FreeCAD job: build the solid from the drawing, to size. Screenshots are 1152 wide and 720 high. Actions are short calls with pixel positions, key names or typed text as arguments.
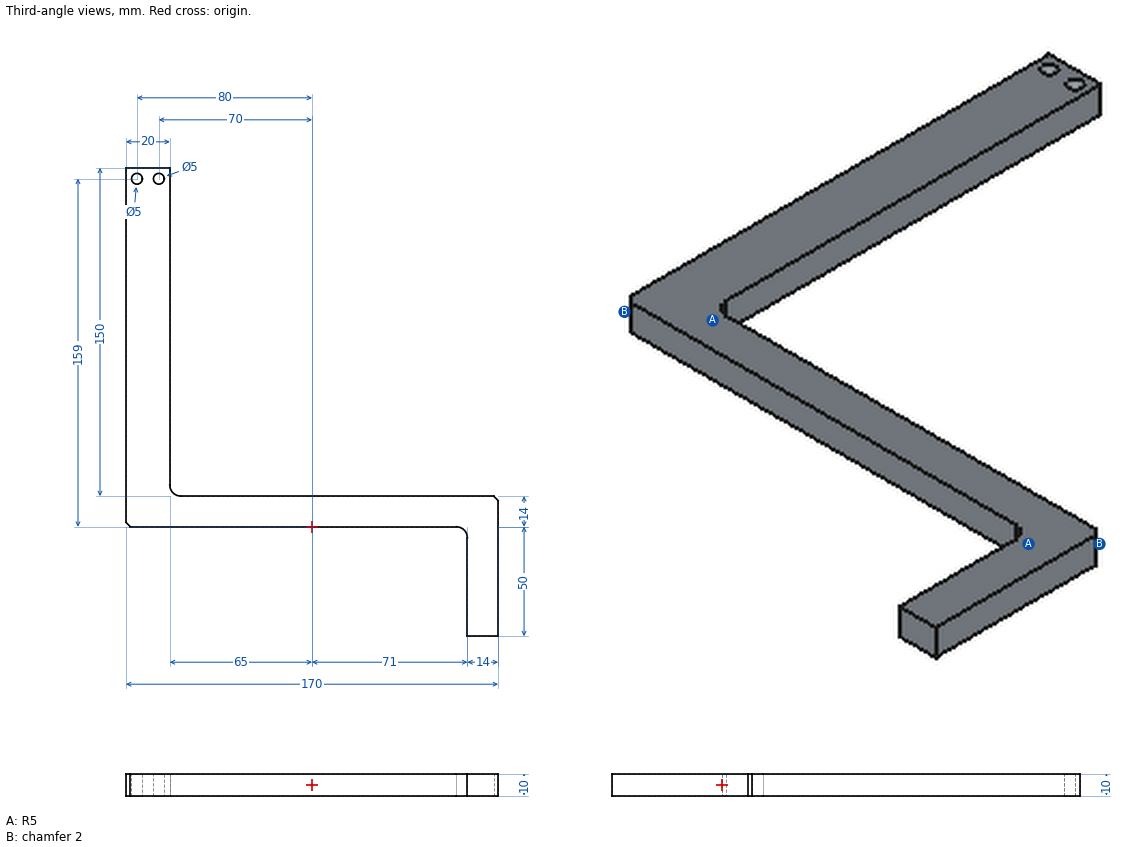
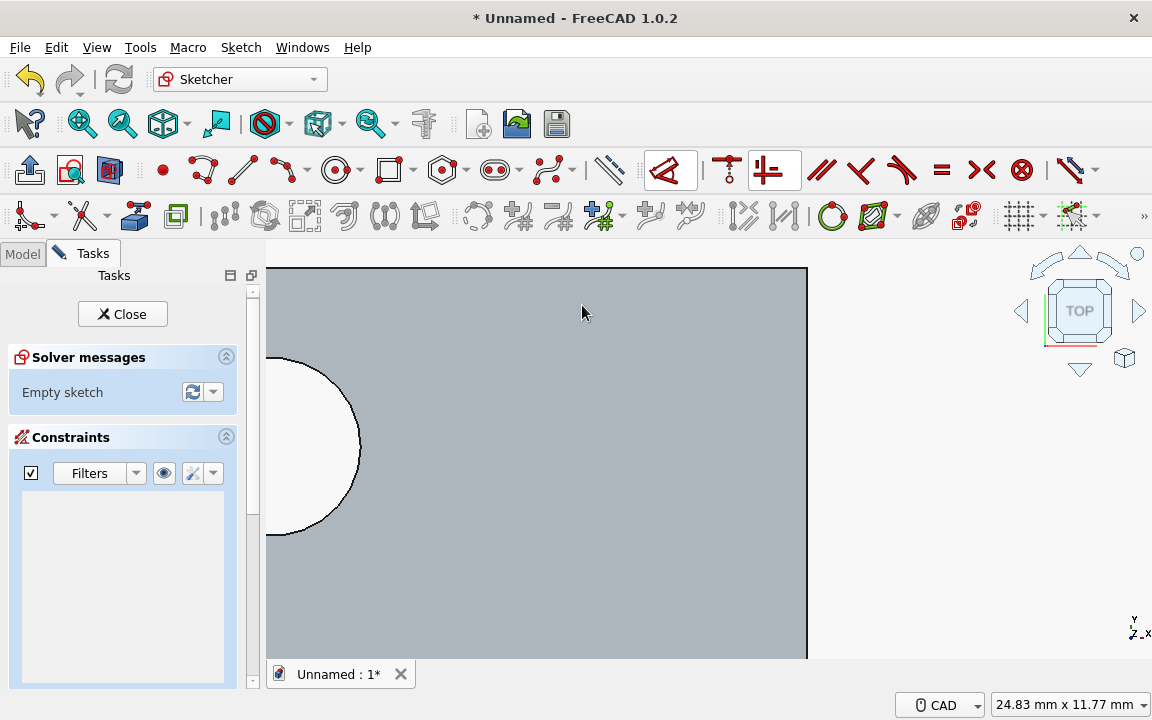
scroll(604, 442, up, 2)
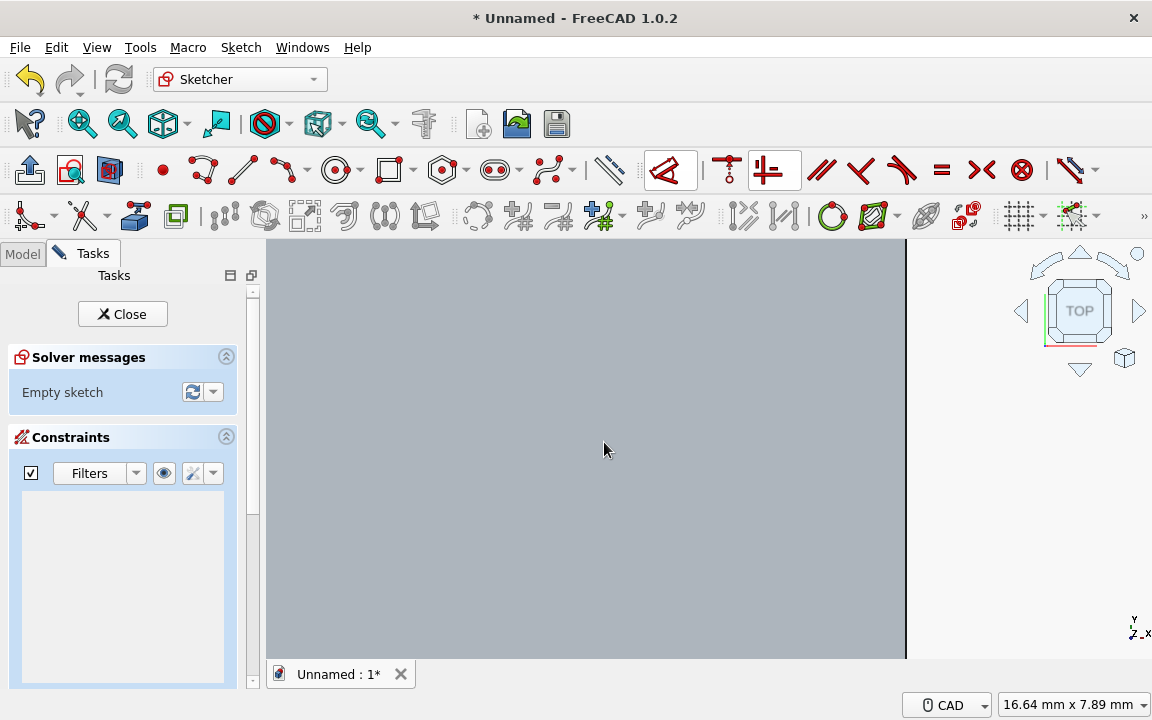
click(336, 170)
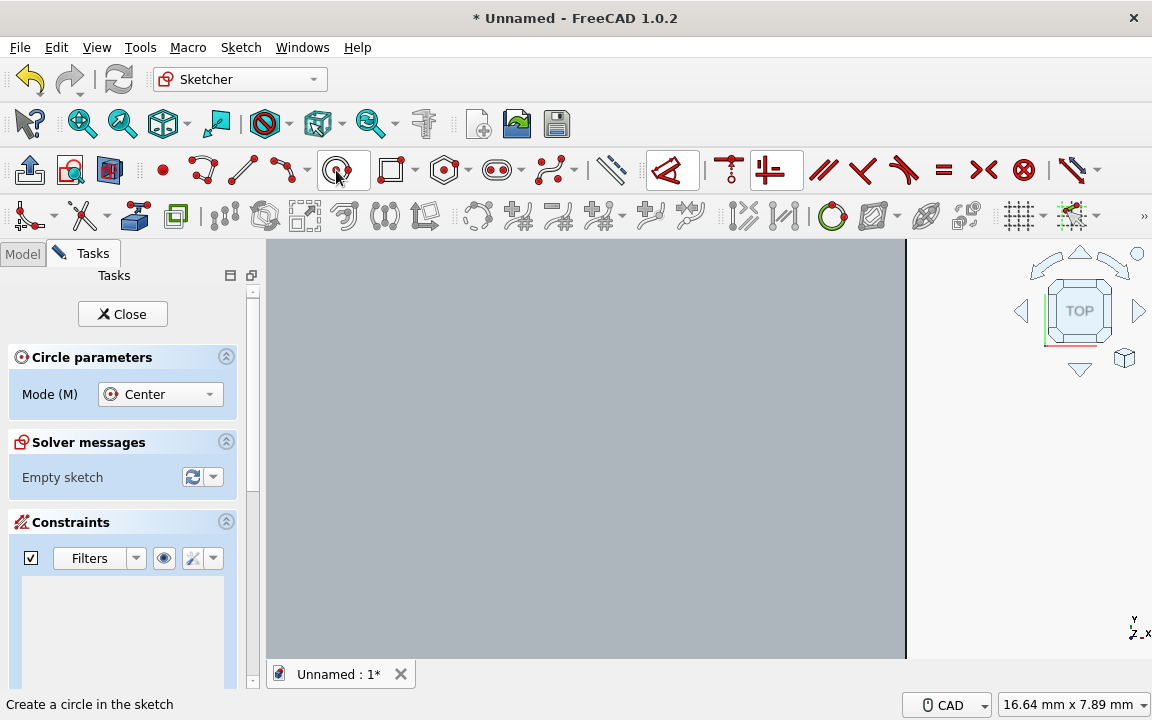
click(640, 449)
move(734, 355)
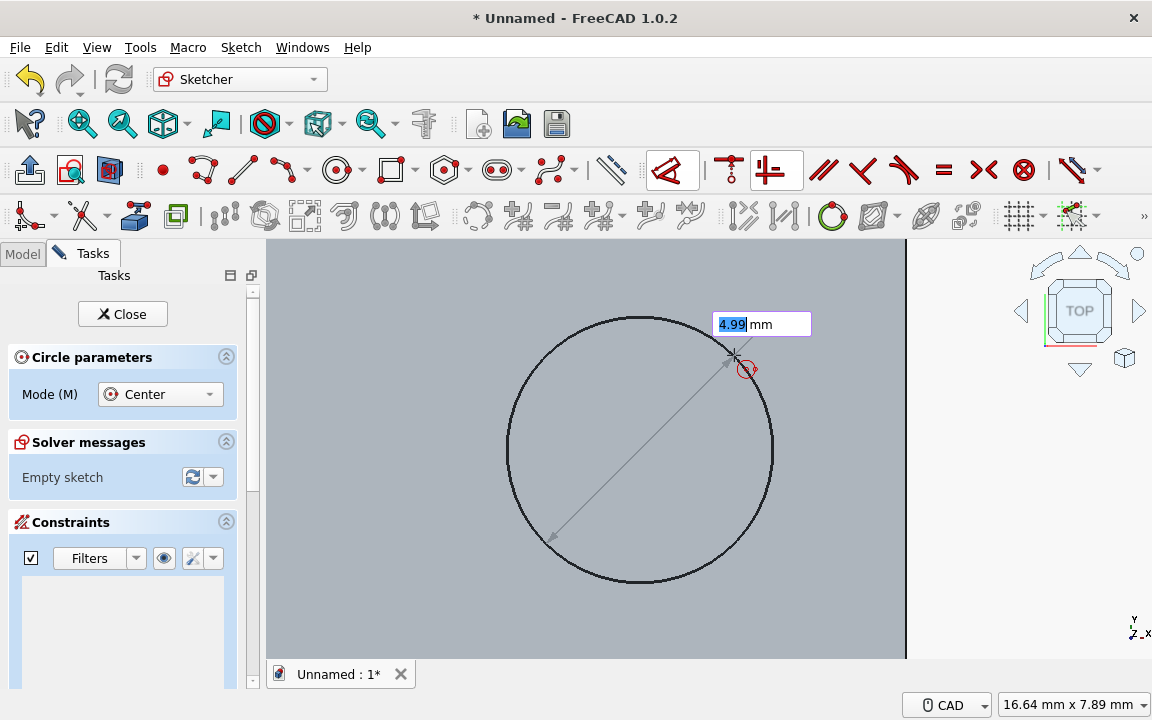
text(5)
key(Return)
key(Escape)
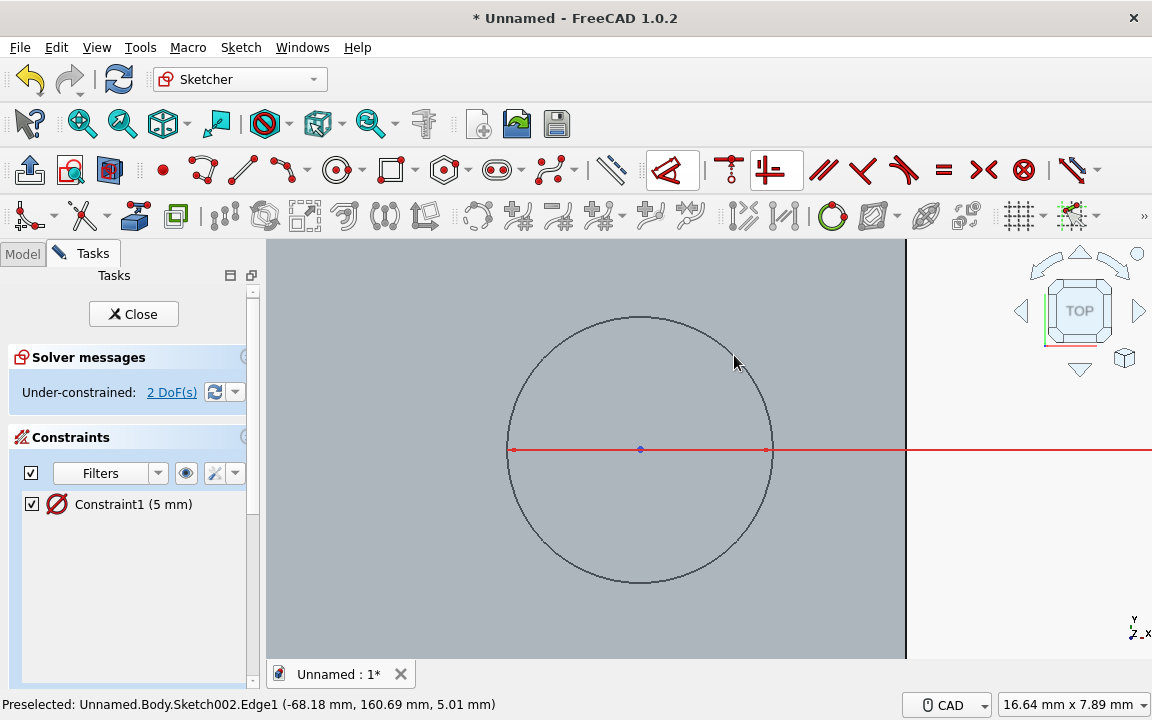
key(d)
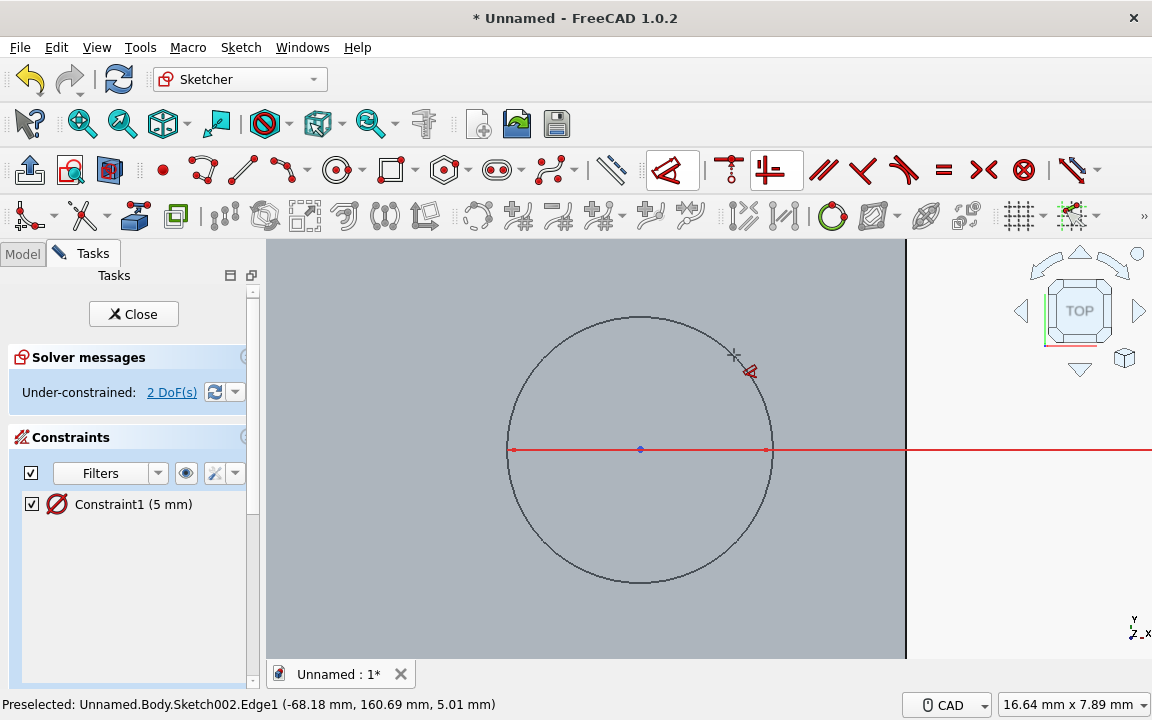
click(640, 450)
click(814, 416)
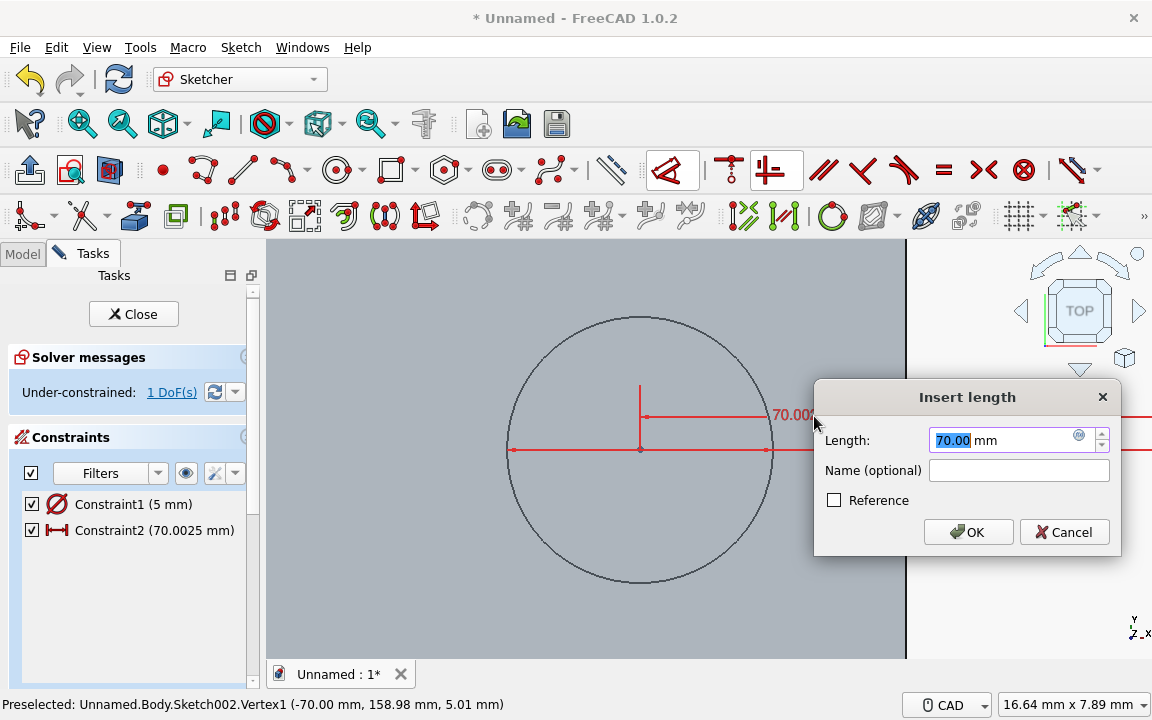
text(70)
key(Return)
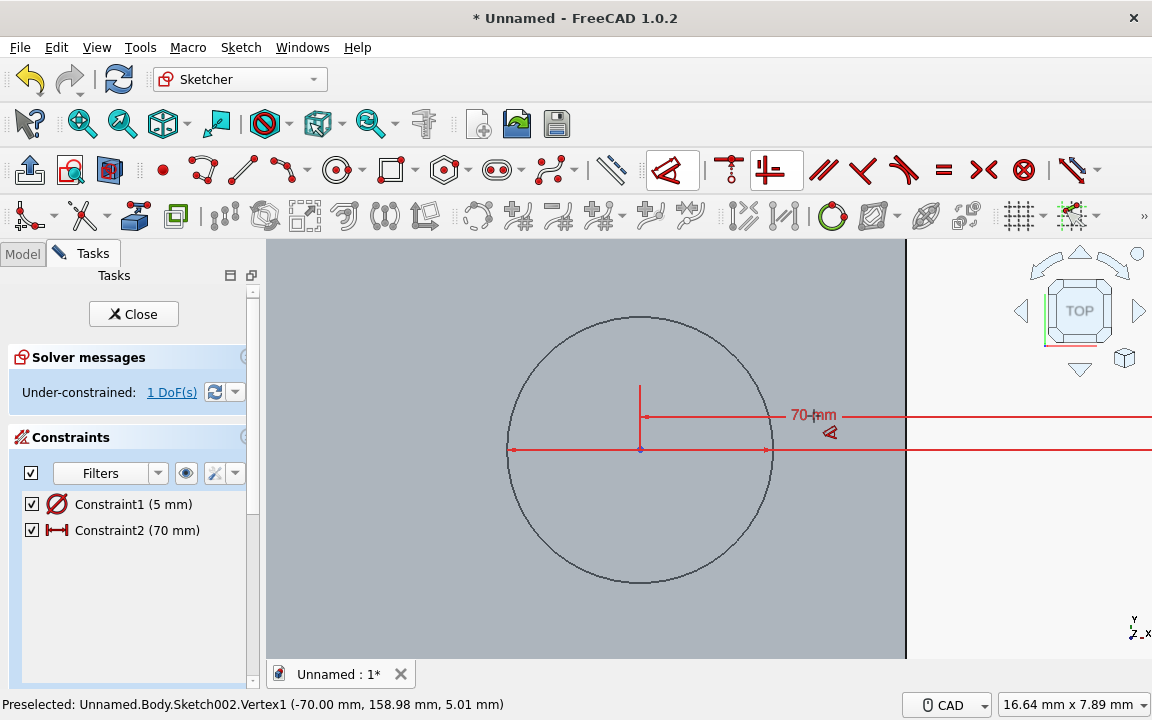
click(640, 450)
click(606, 540)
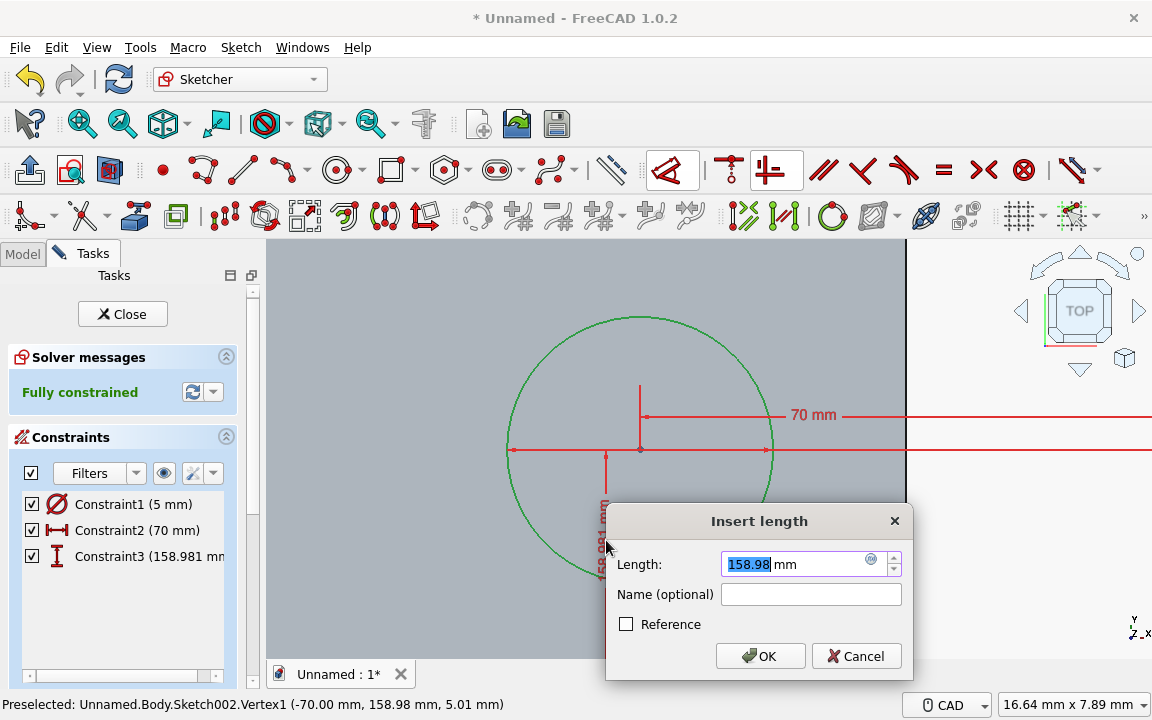
text(159)
key(Return)
key(Escape)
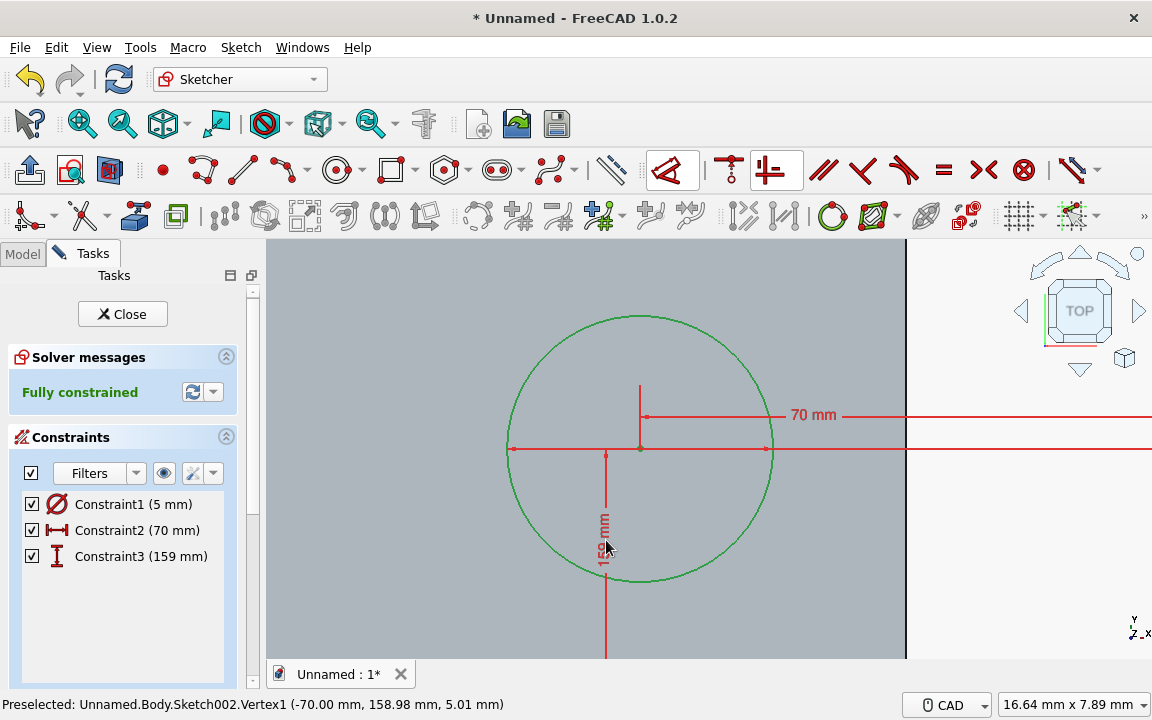
click(123, 314)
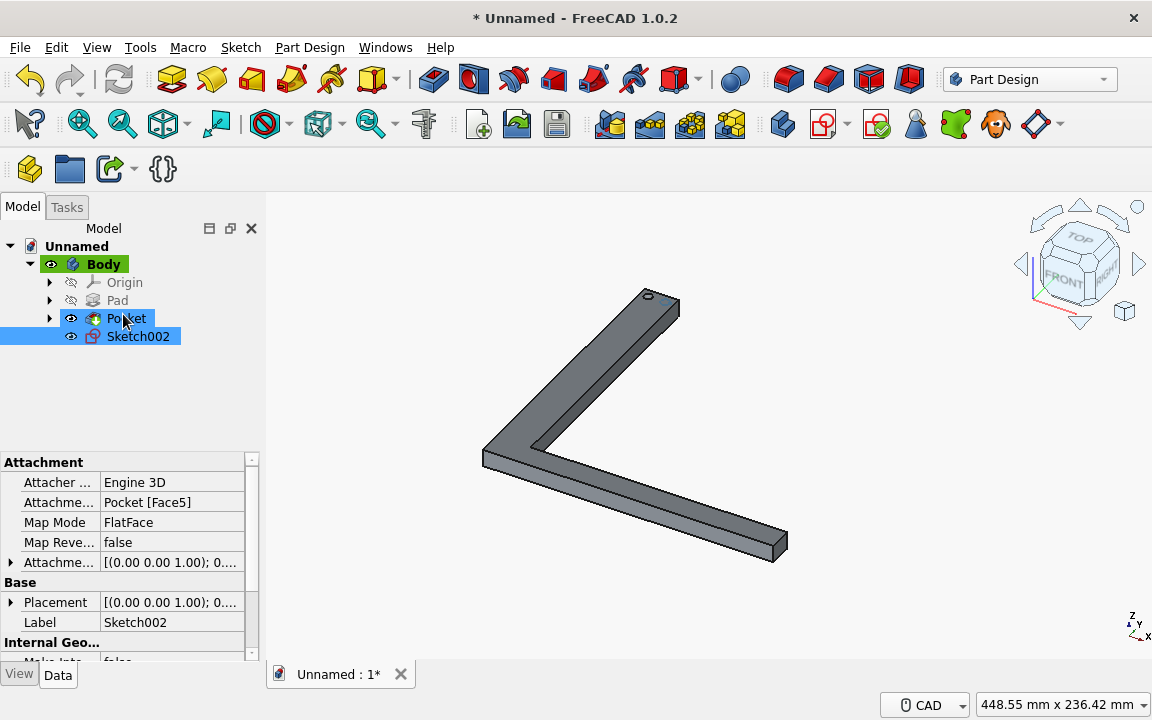
click(434, 80)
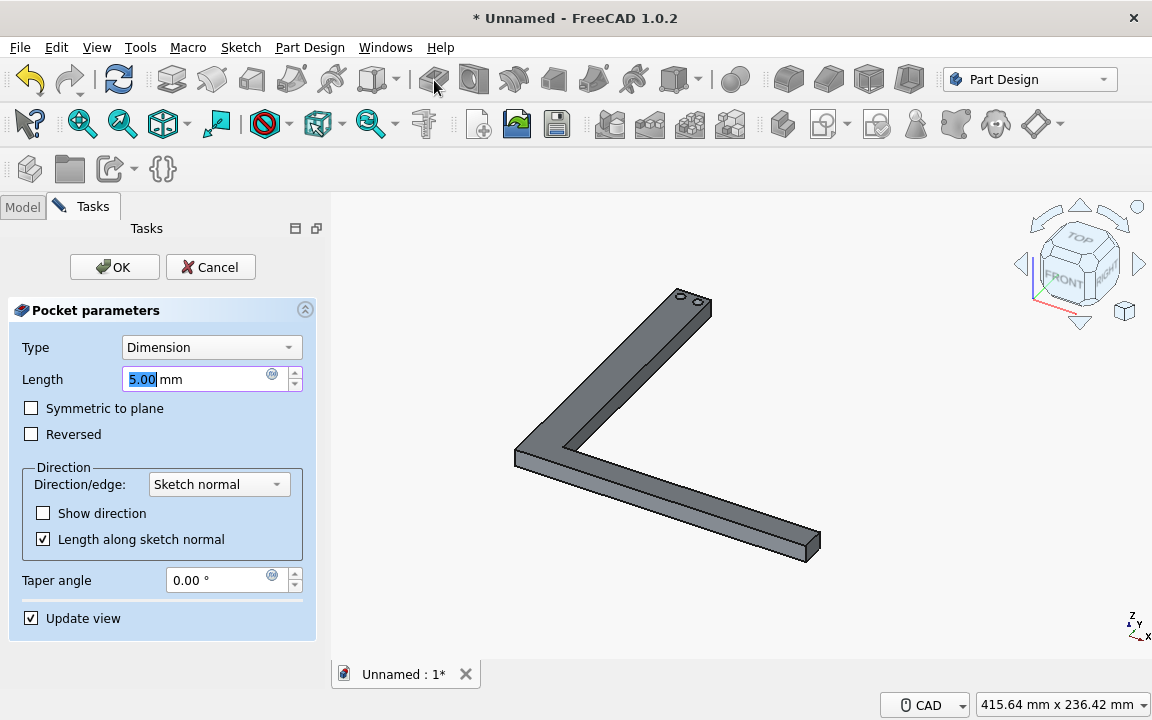
click(212, 348)